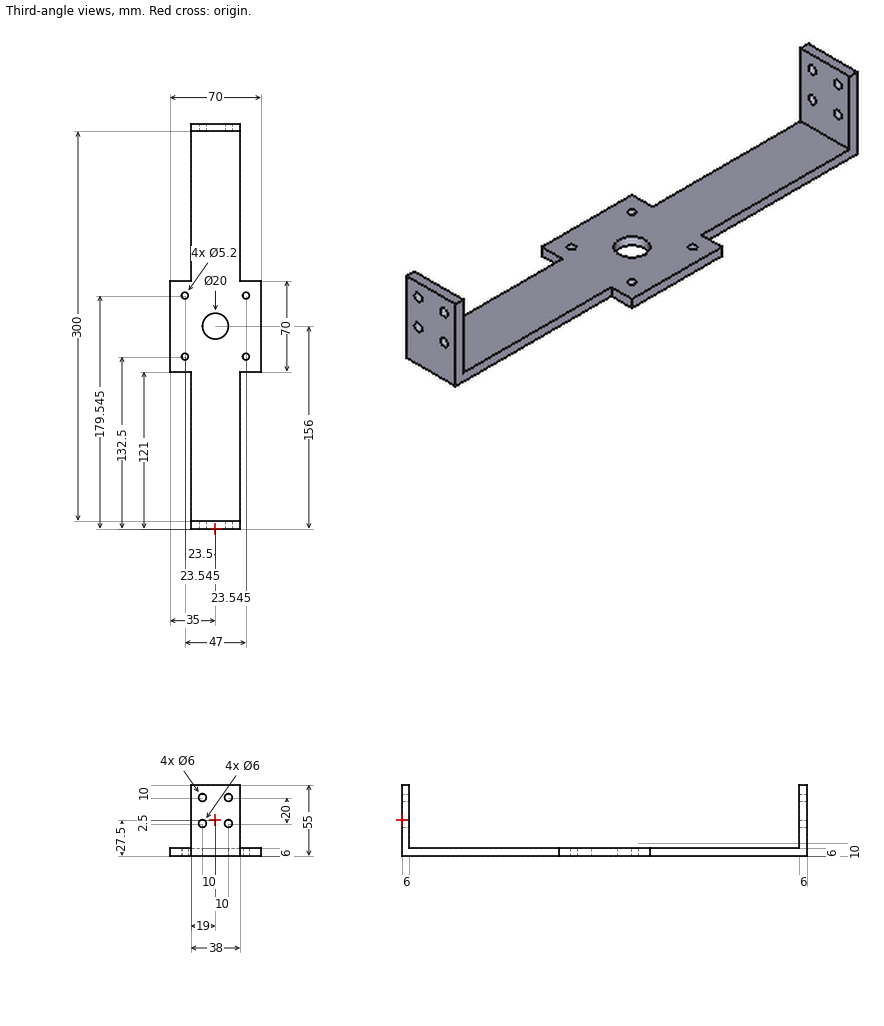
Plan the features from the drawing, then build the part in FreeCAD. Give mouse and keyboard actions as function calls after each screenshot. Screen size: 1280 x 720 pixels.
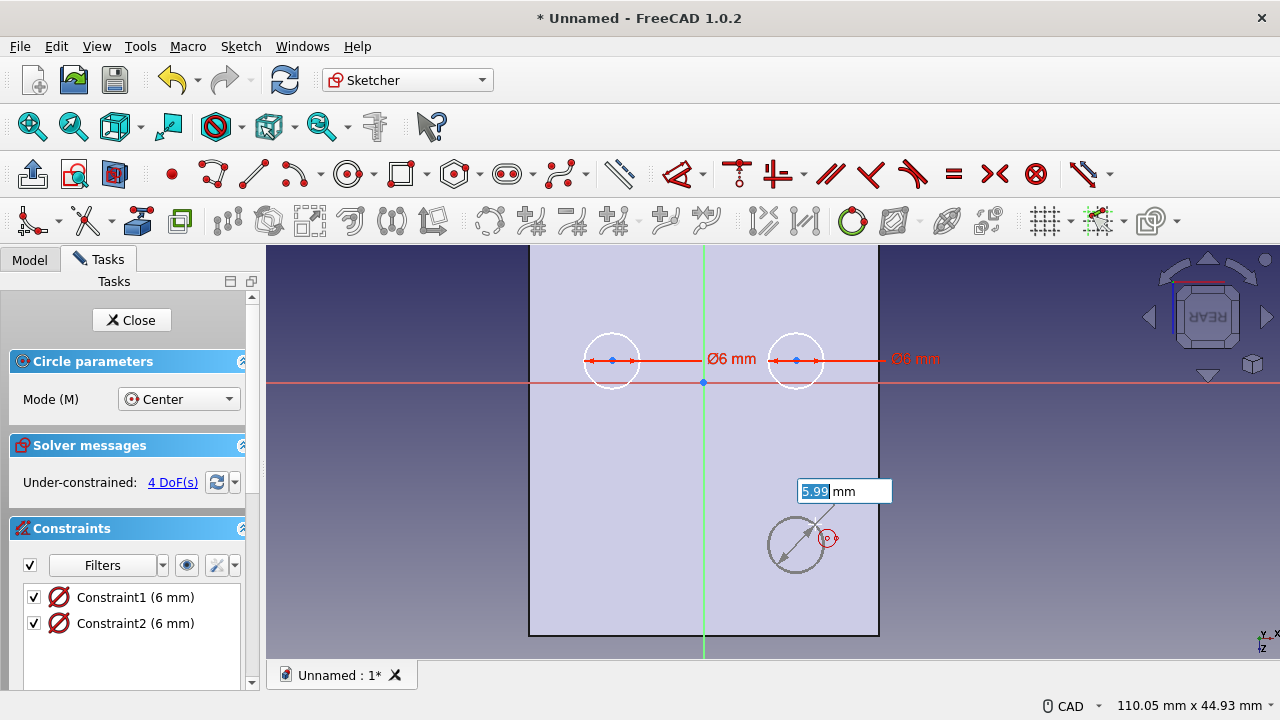
text(6)
key(Return)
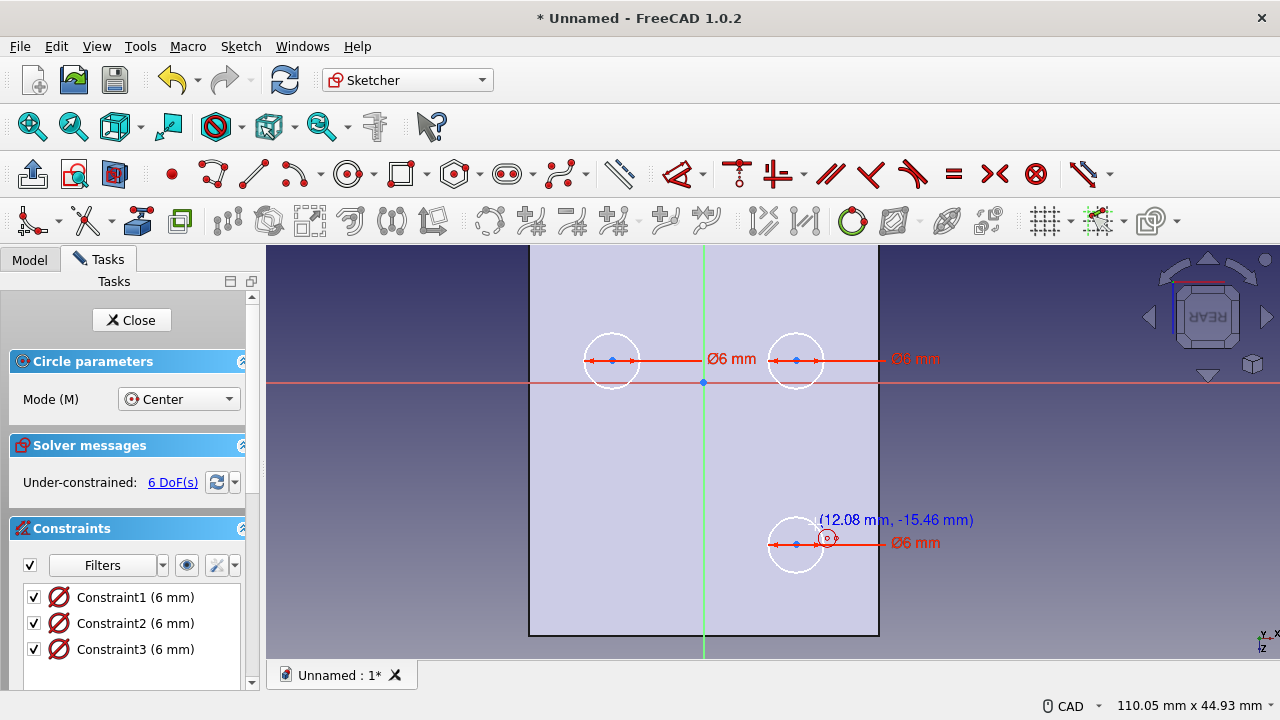
click(612, 544)
move(631, 524)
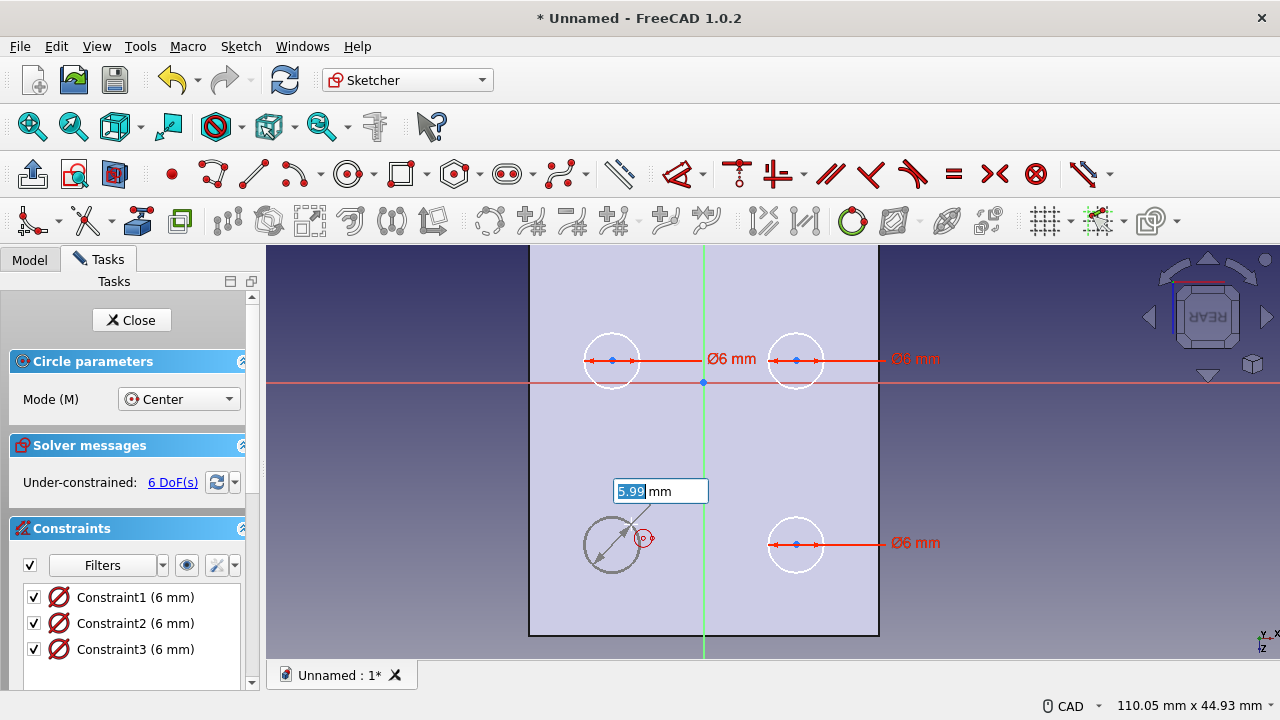
text(6)
key(Return)
key(Escape)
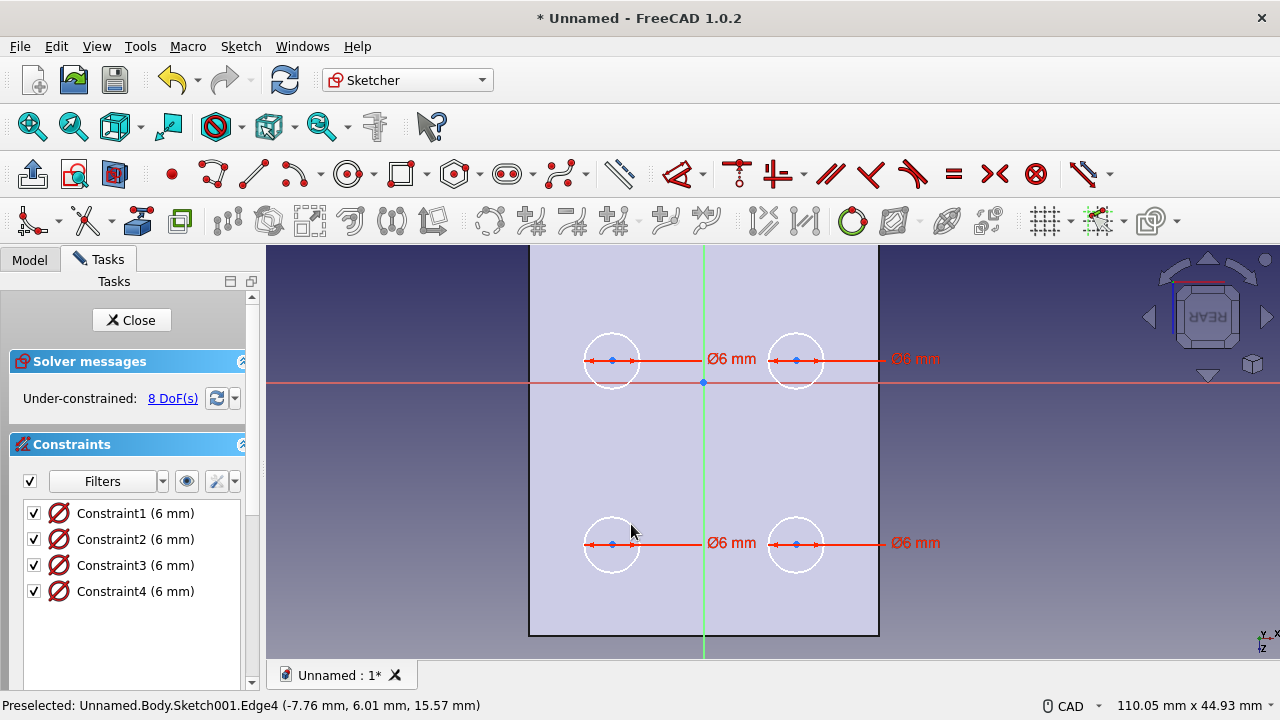
click(612, 361)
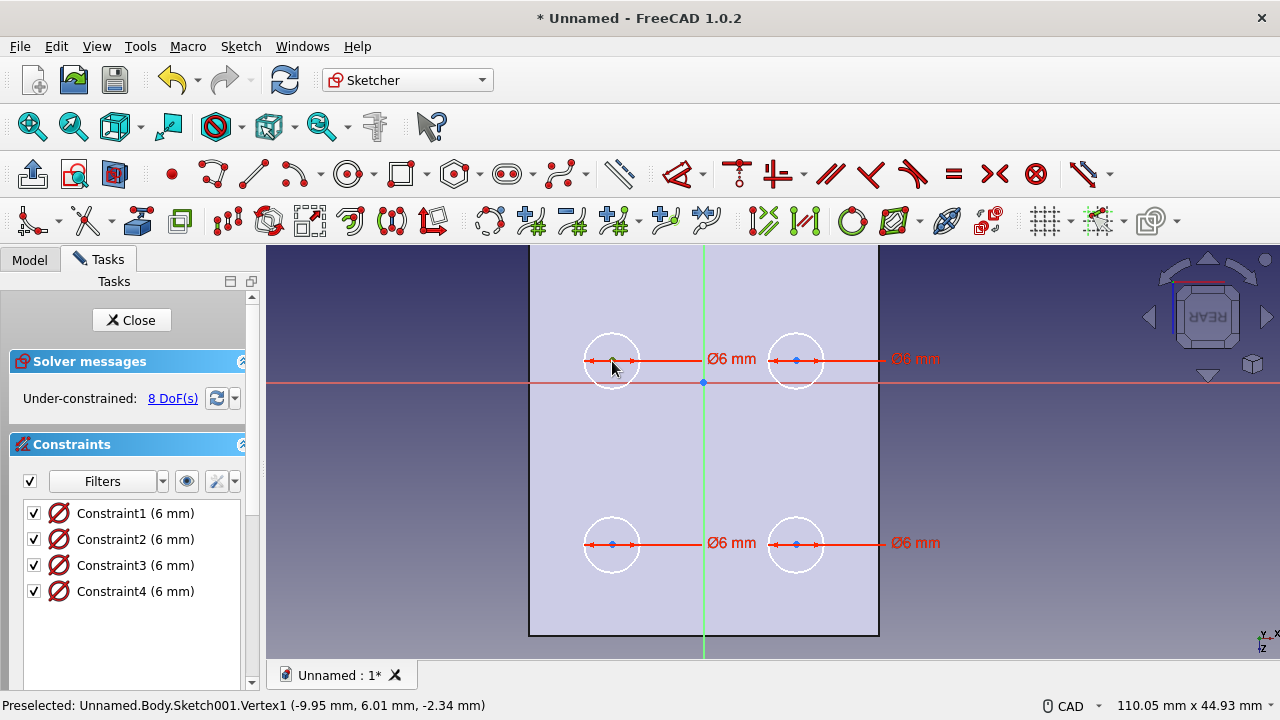
click(796, 361)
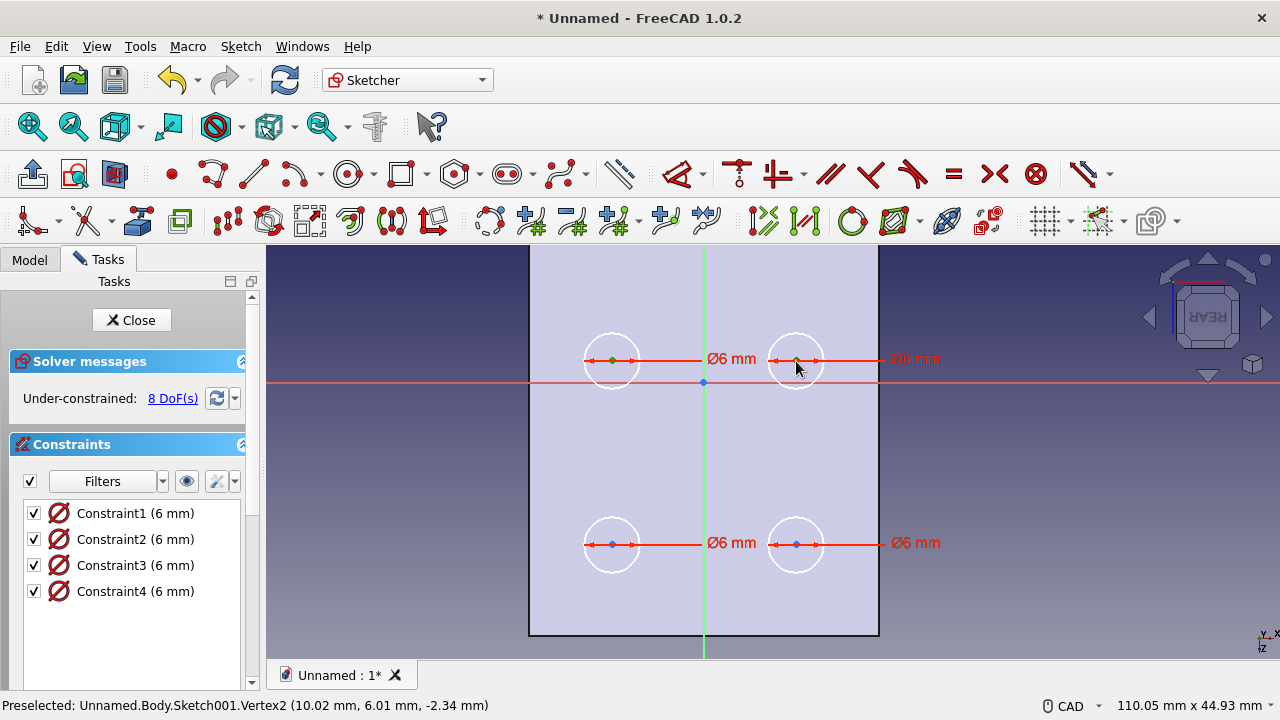
click(804, 174)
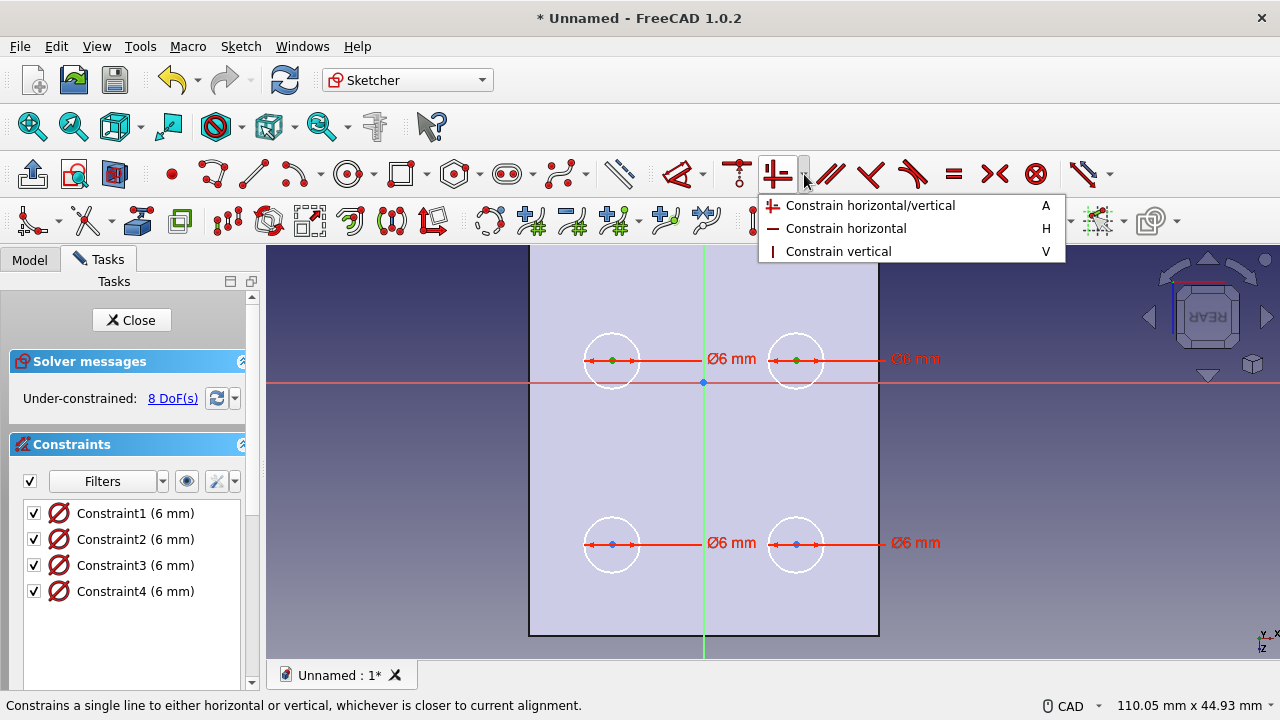
click(912, 228)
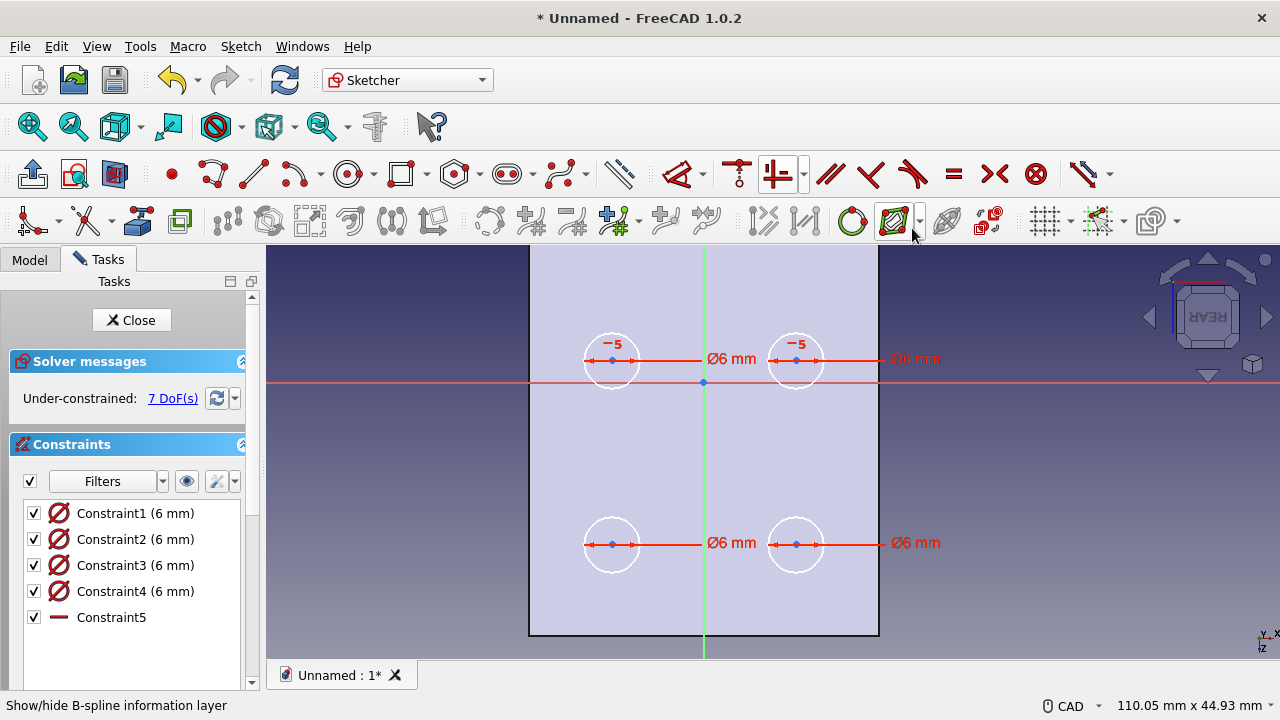
click(796, 361)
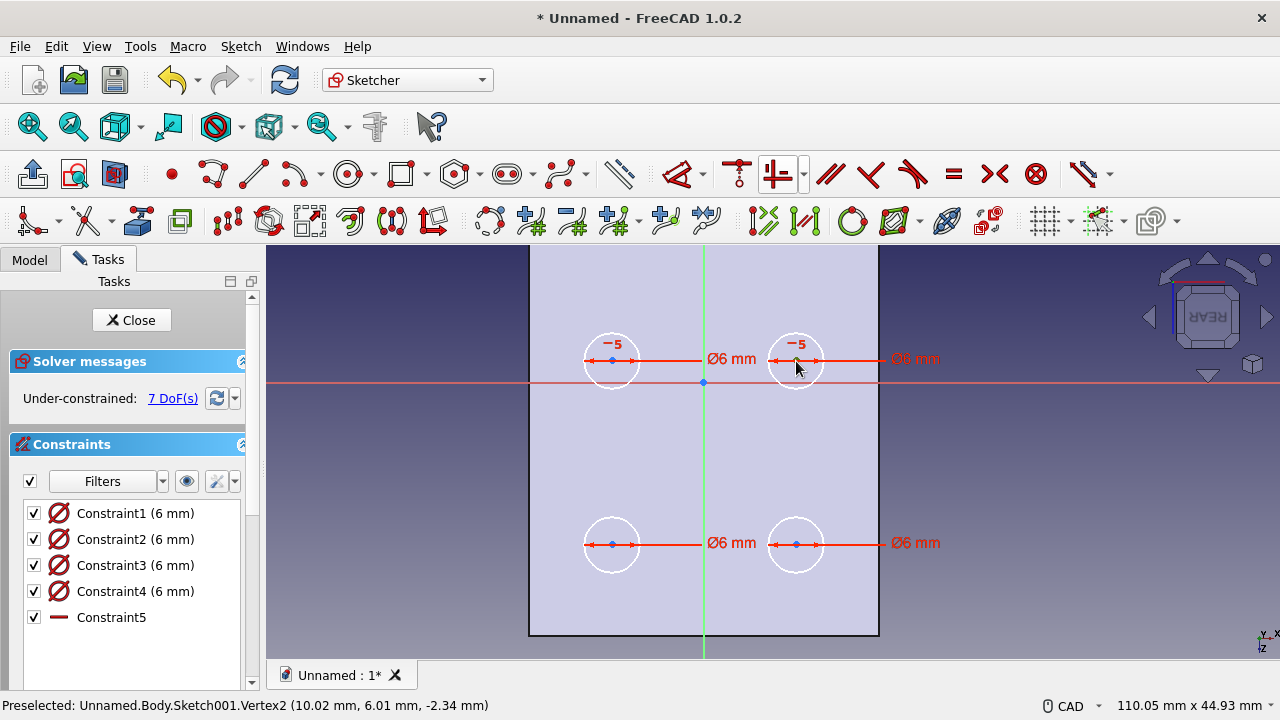
click(796, 545)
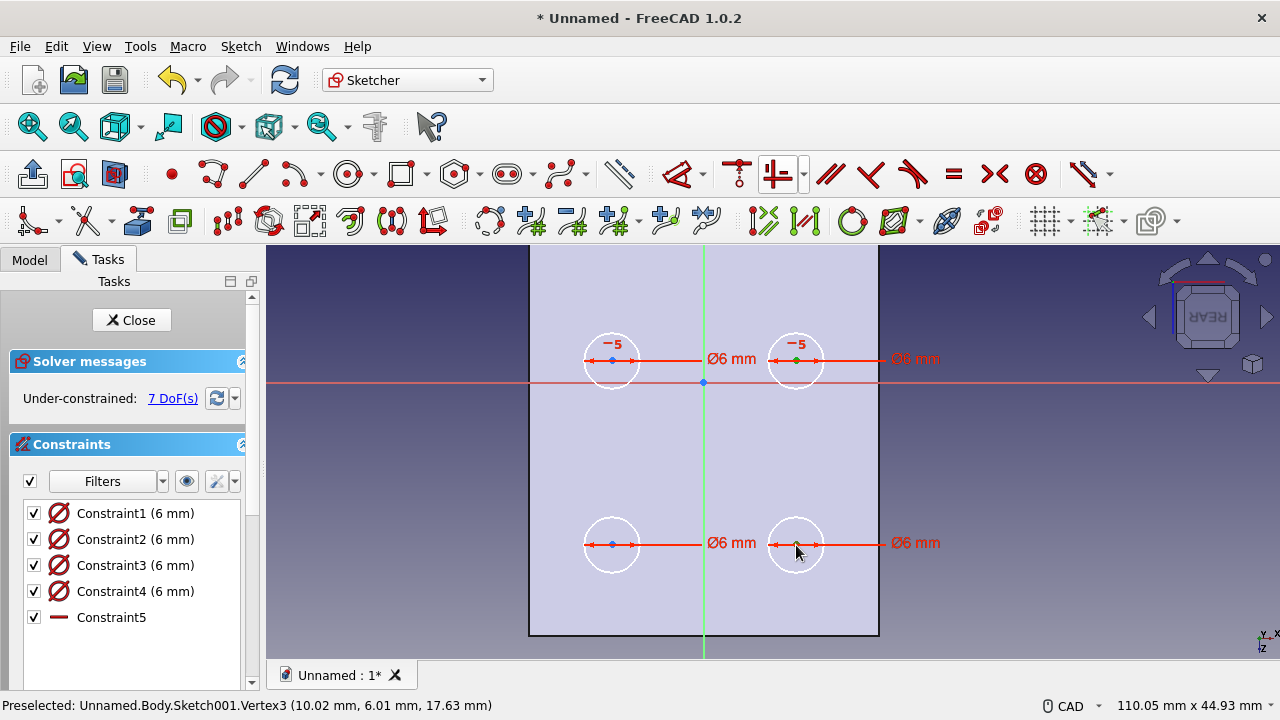
click(804, 174)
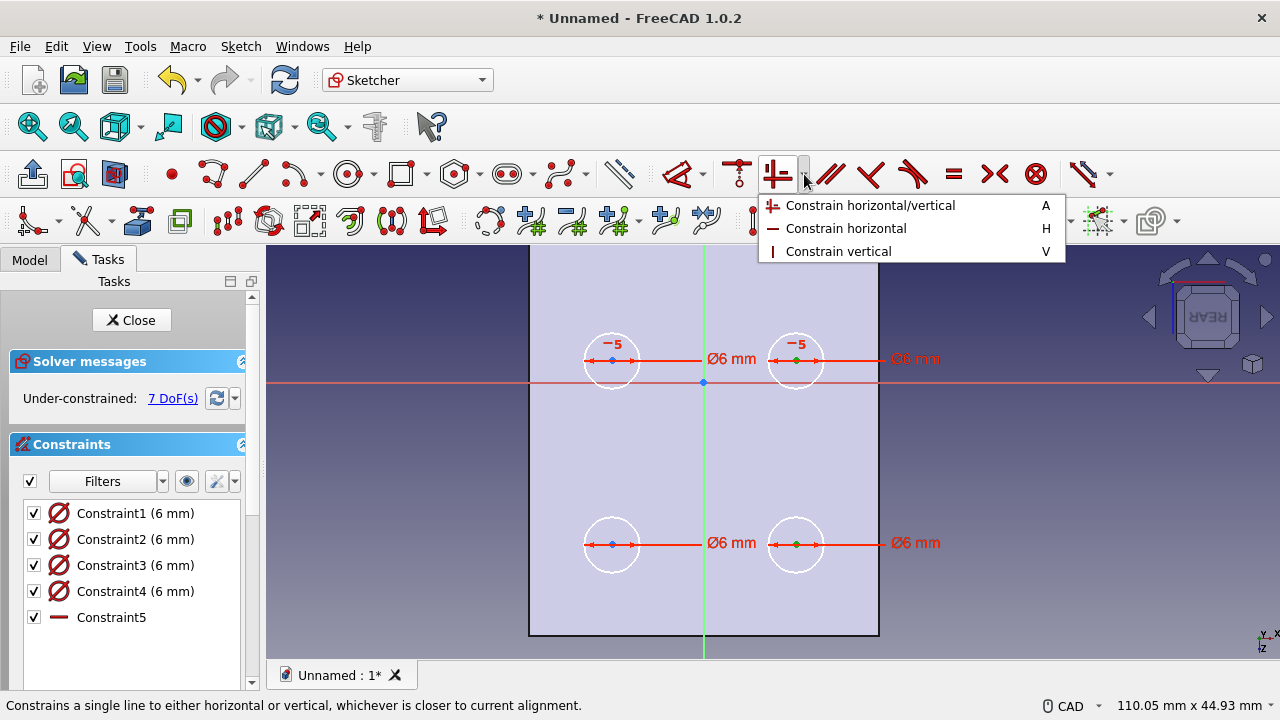
click(912, 252)